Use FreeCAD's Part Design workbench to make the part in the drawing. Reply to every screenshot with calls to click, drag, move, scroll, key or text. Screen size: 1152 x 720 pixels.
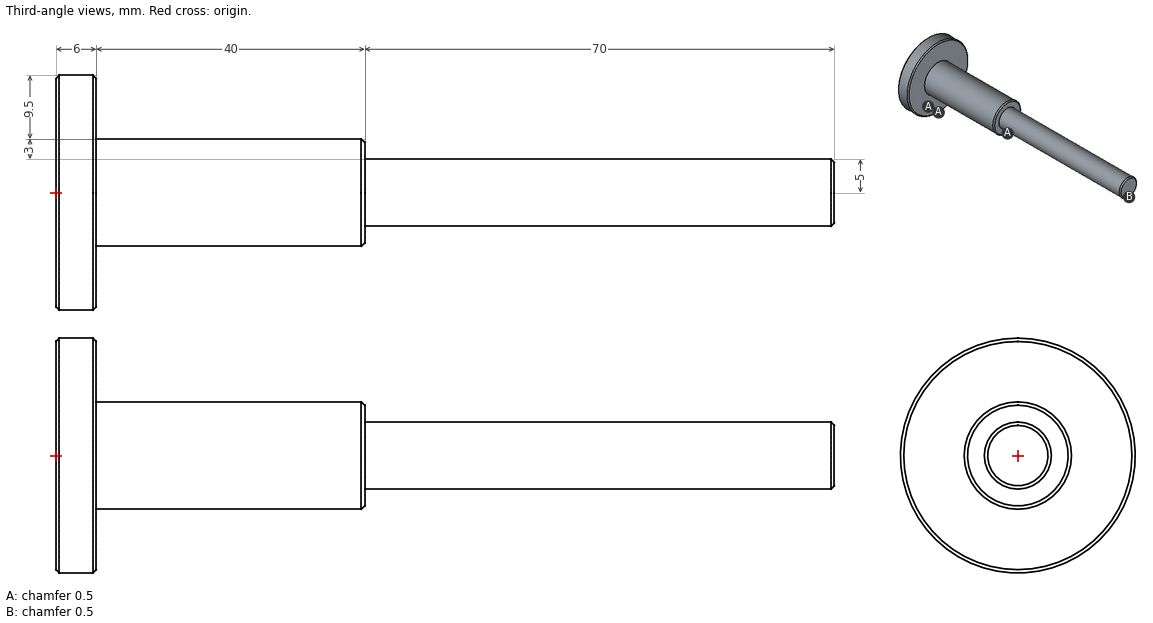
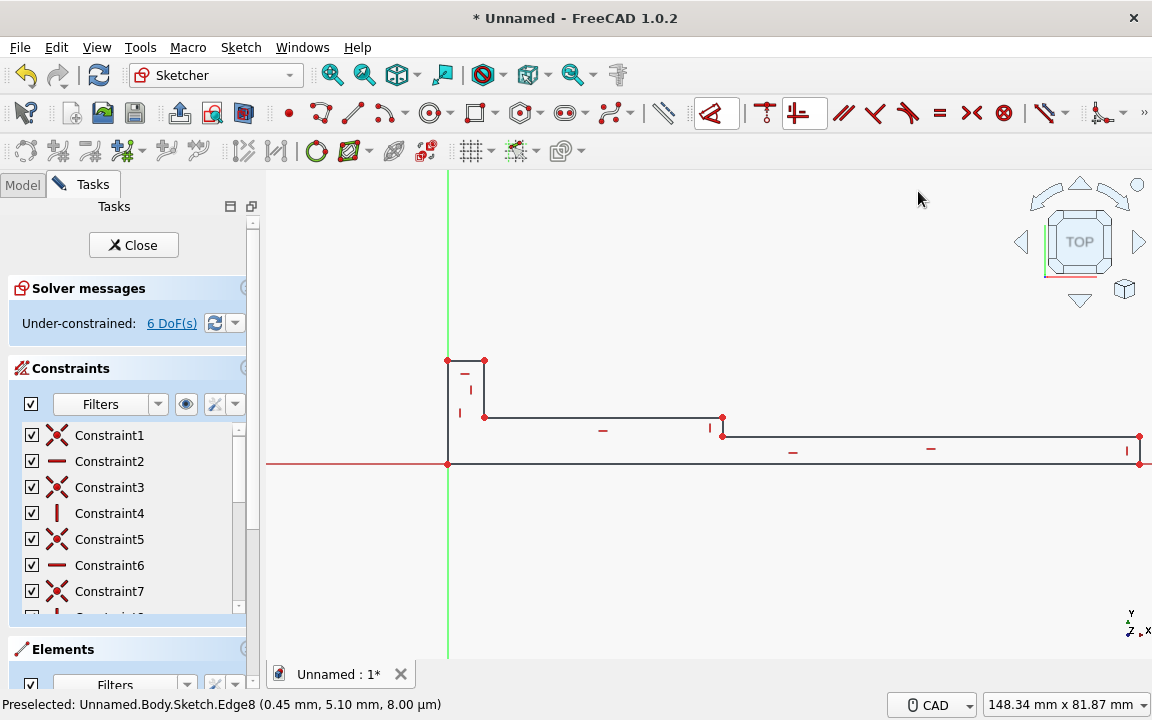
click(710, 114)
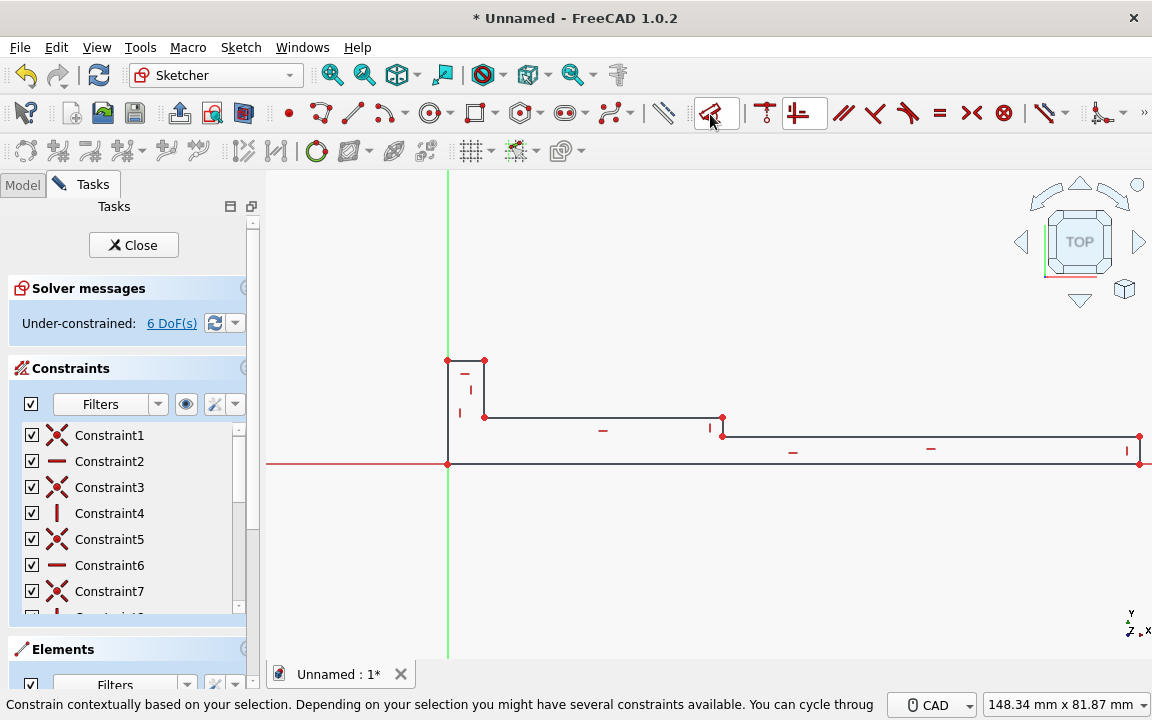
scroll(328, 419, down, 2)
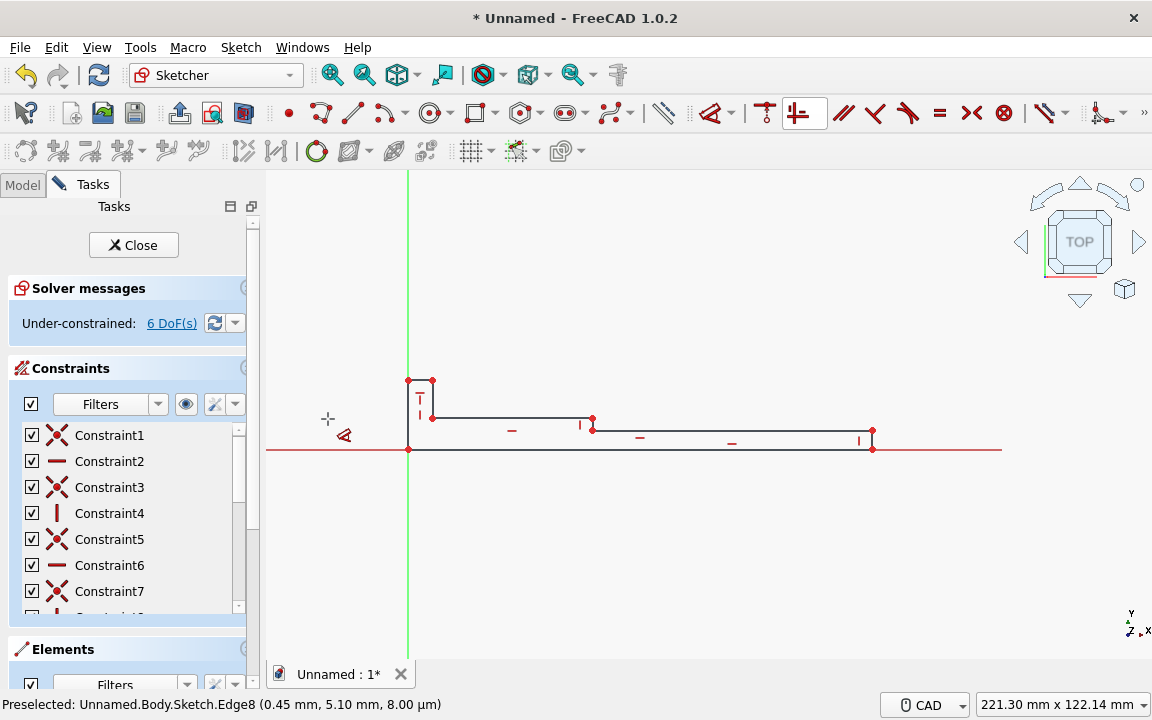
scroll(872, 442, up, 4)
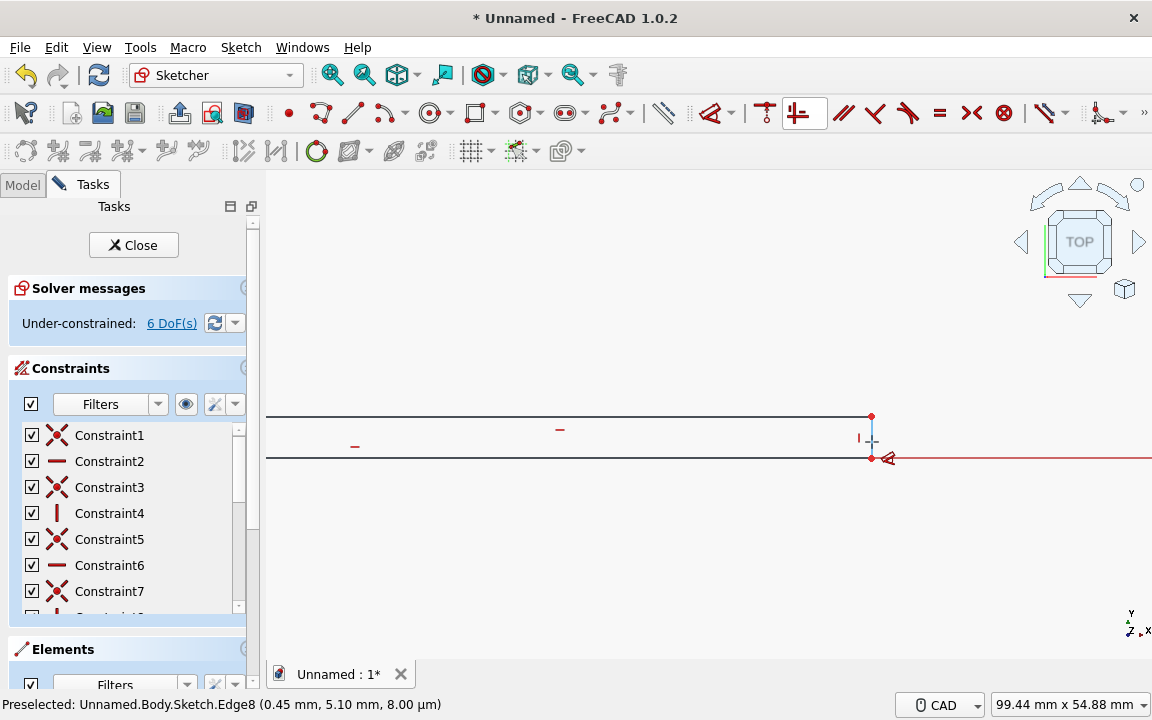
click(872, 442)
click(906, 438)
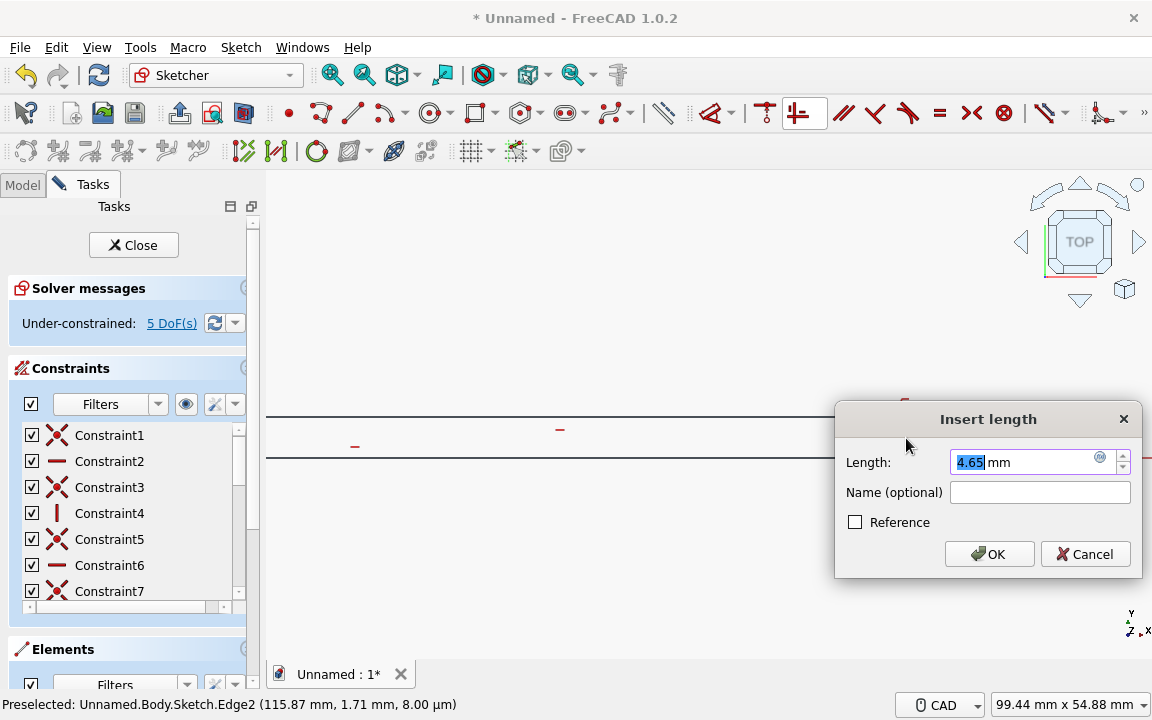
text(5)
key(Return)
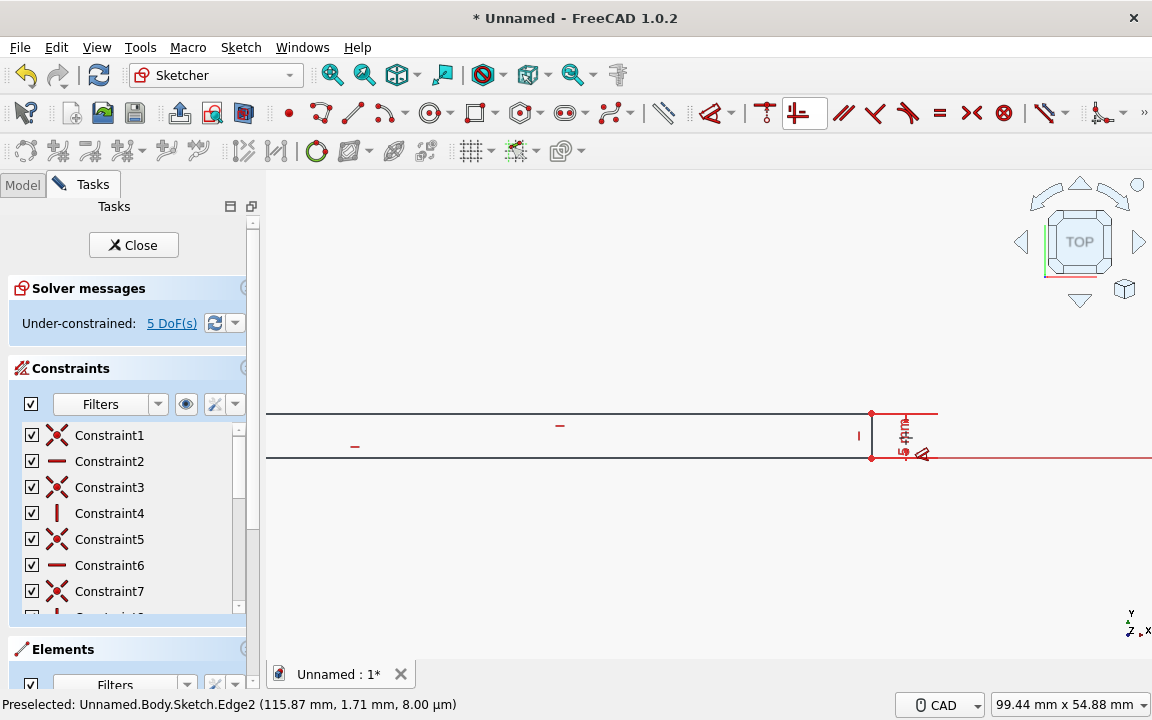
scroll(873, 442, down, 4)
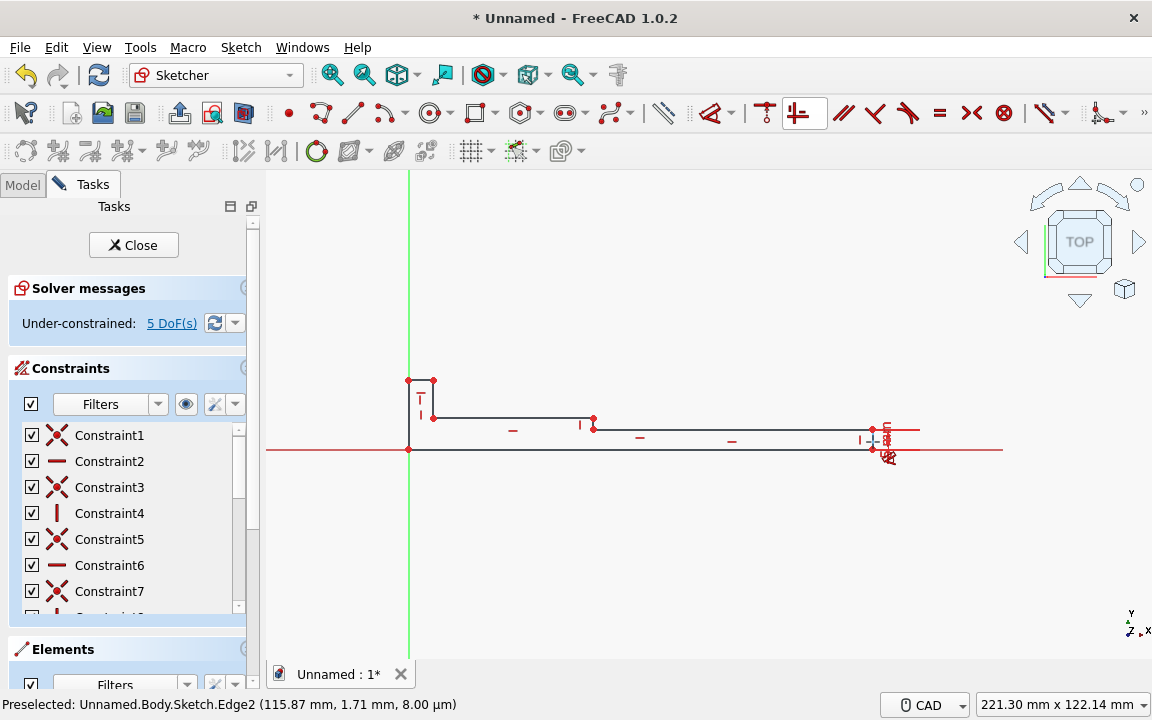
scroll(593, 425, up, 6)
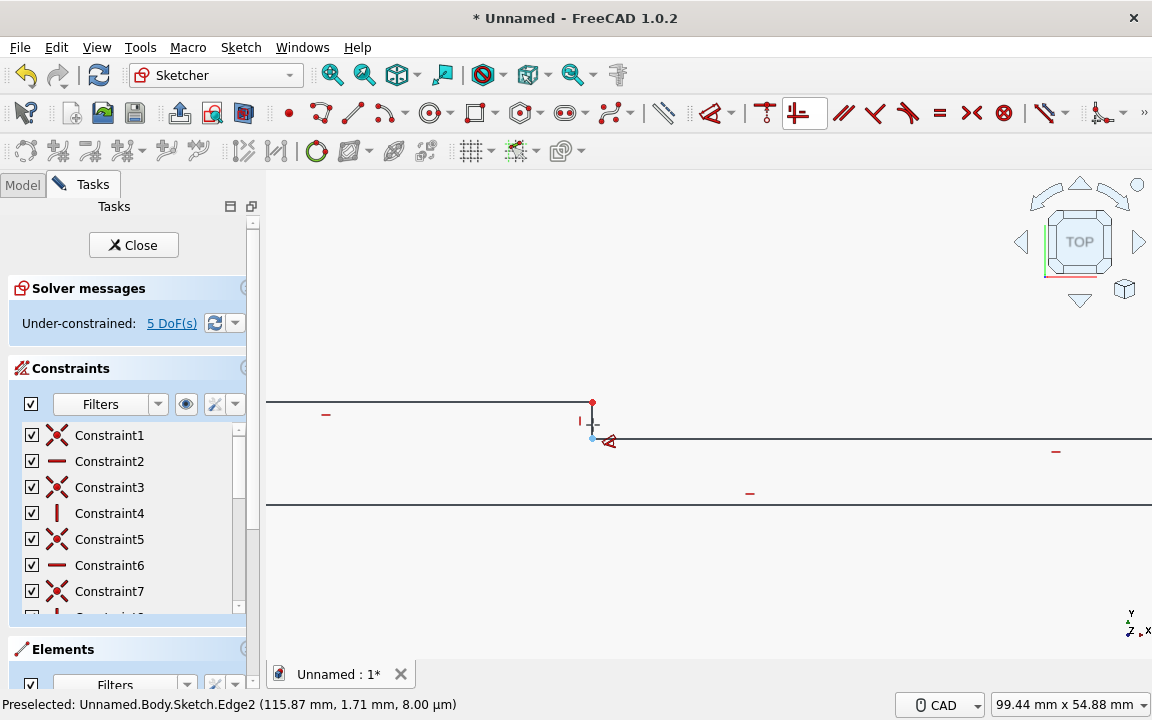
click(592, 424)
click(558, 421)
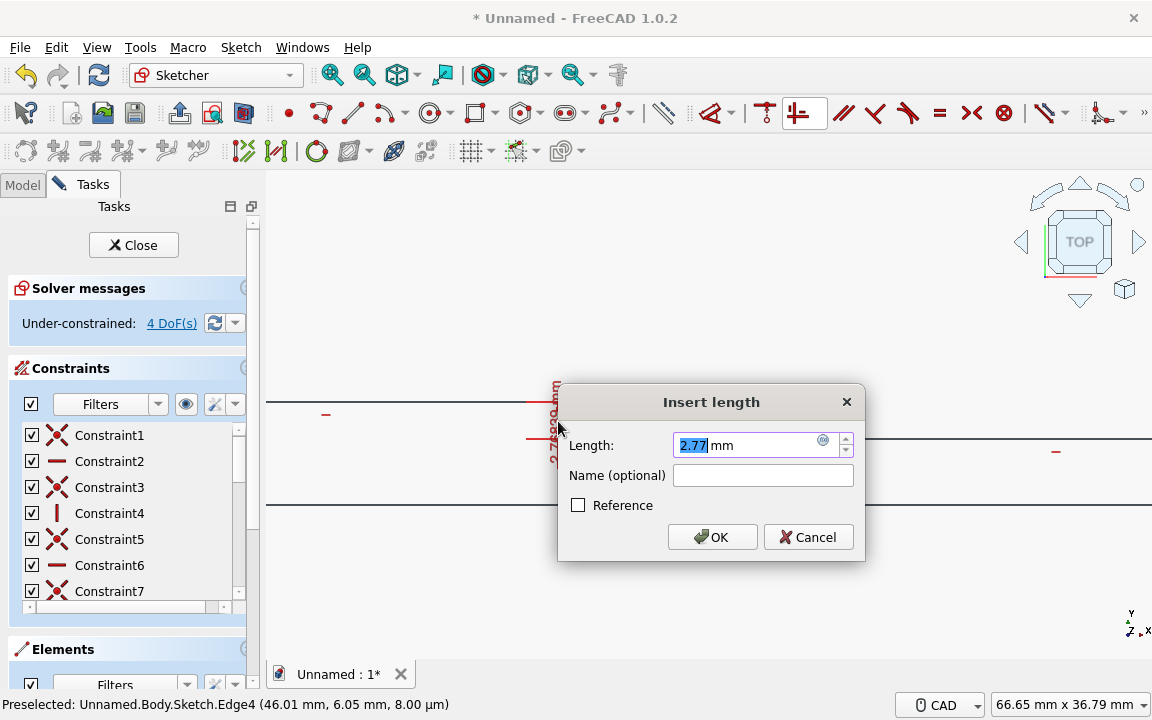
text(3)
key(Return)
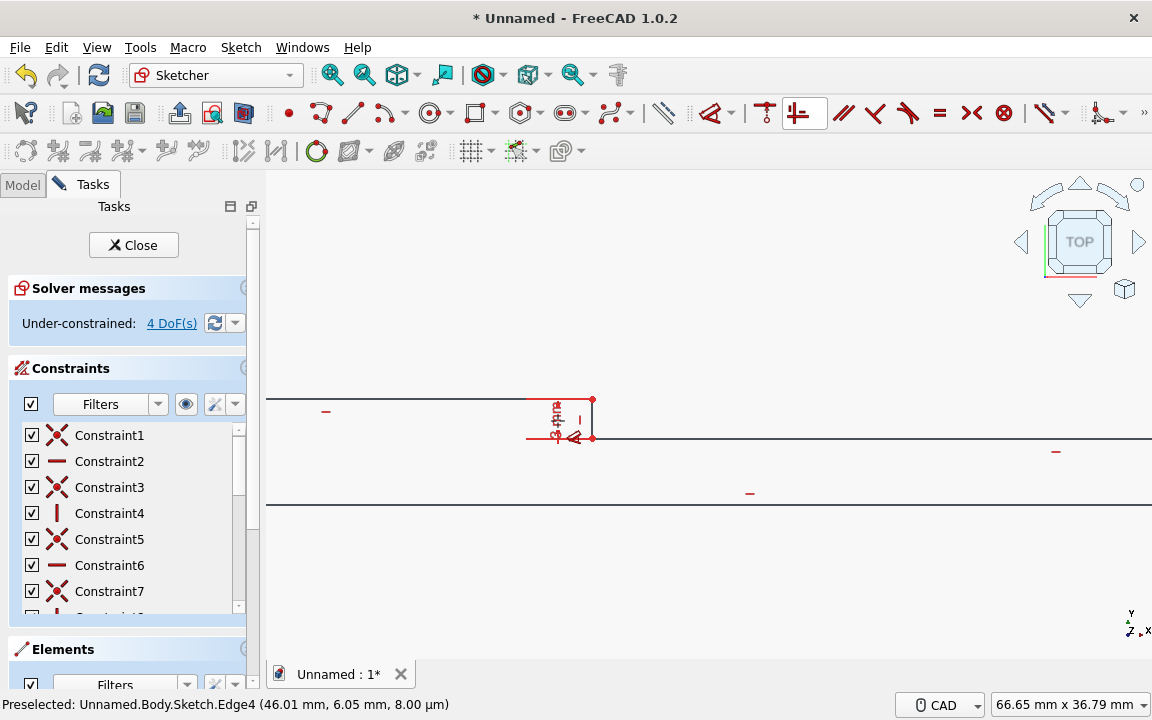
scroll(593, 425, down, 6)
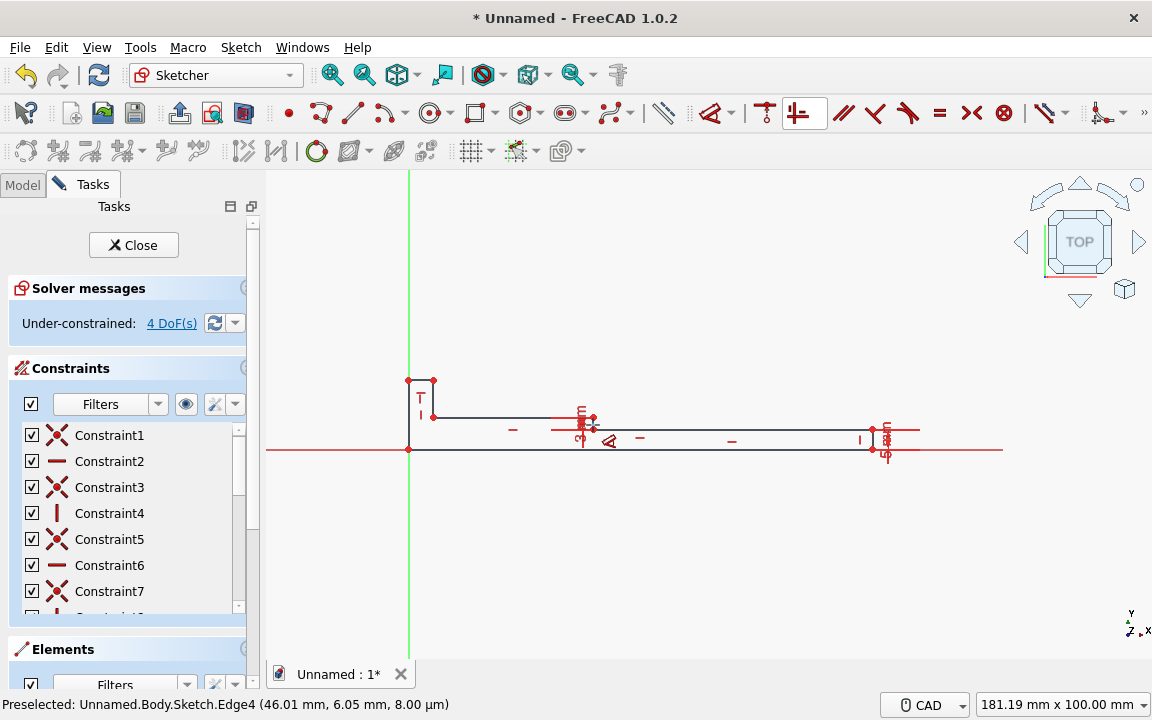
scroll(426, 380, up, 4)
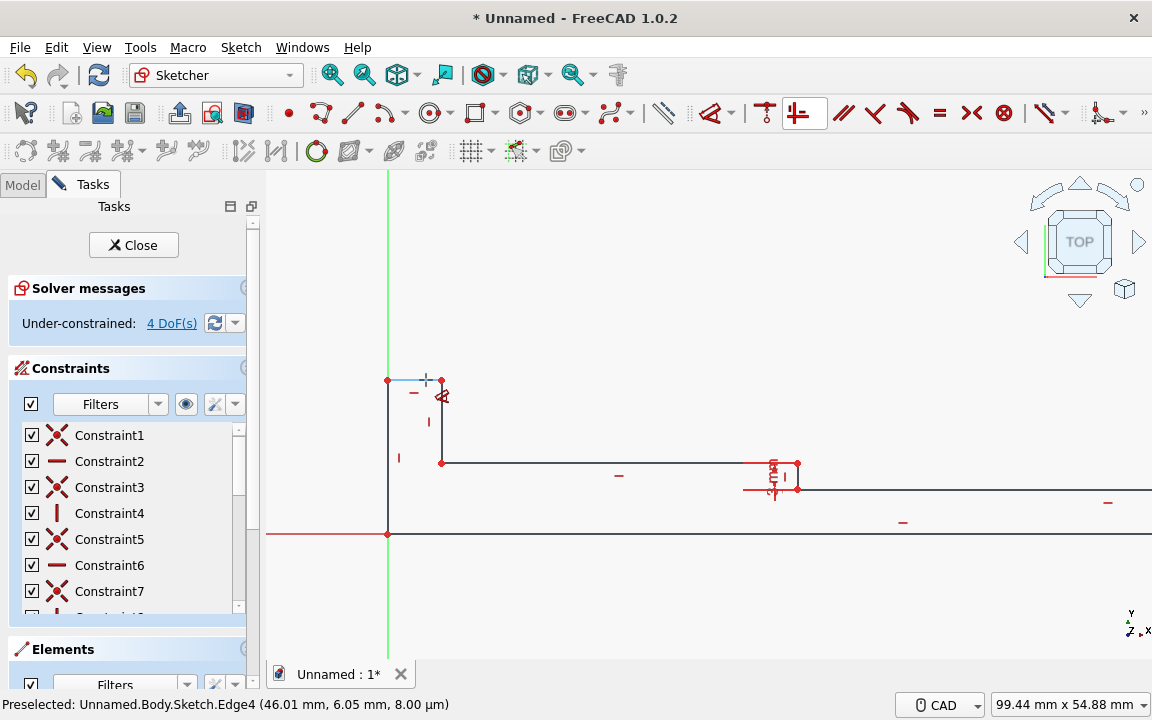
click(425, 380)
click(415, 346)